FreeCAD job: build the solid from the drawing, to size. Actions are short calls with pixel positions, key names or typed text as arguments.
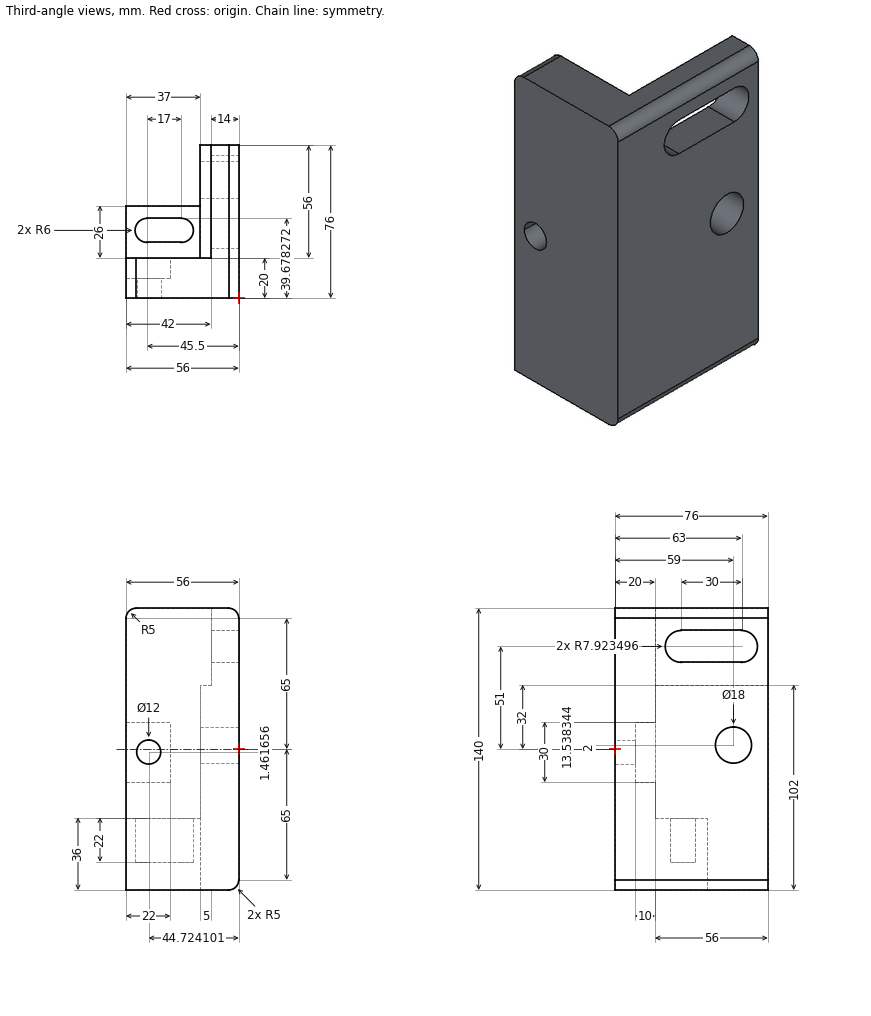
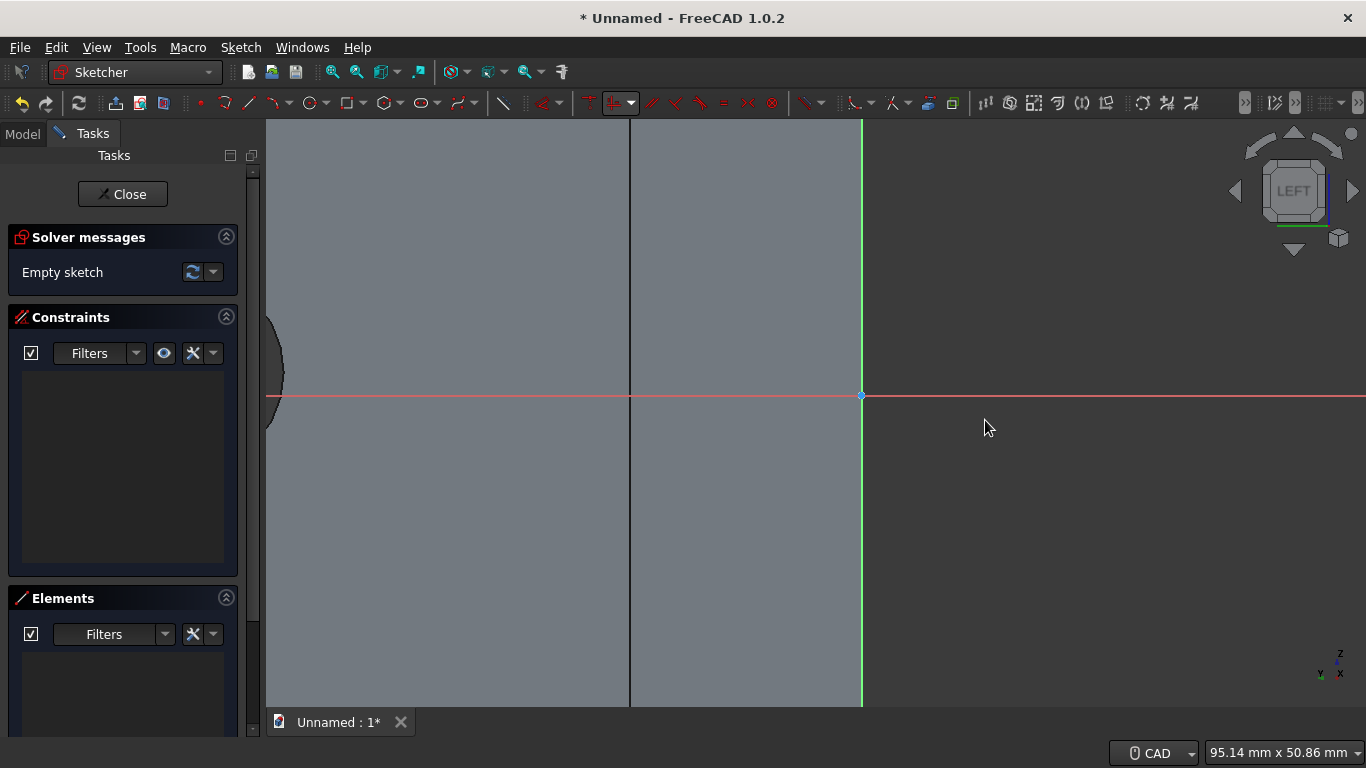
key(g)
key(r)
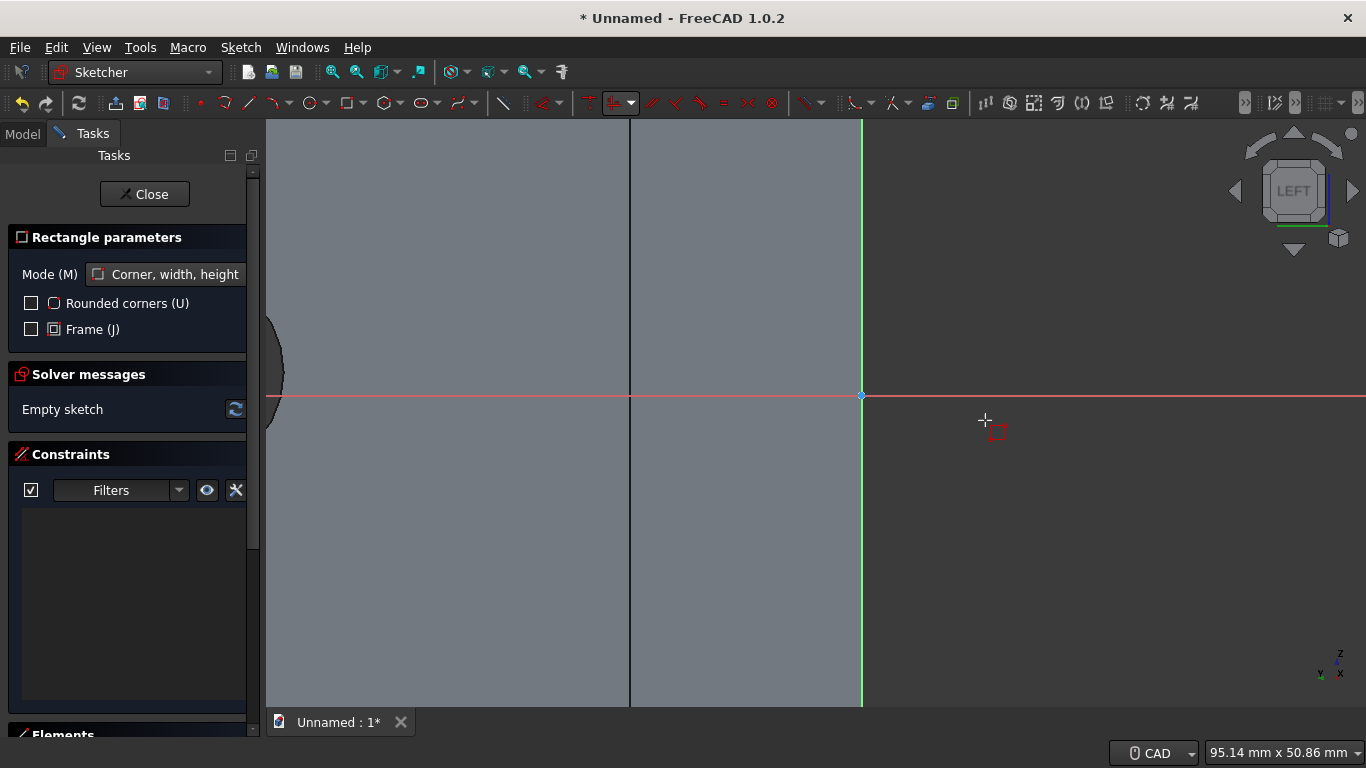
click(630, 239)
click(746, 586)
key(Escape)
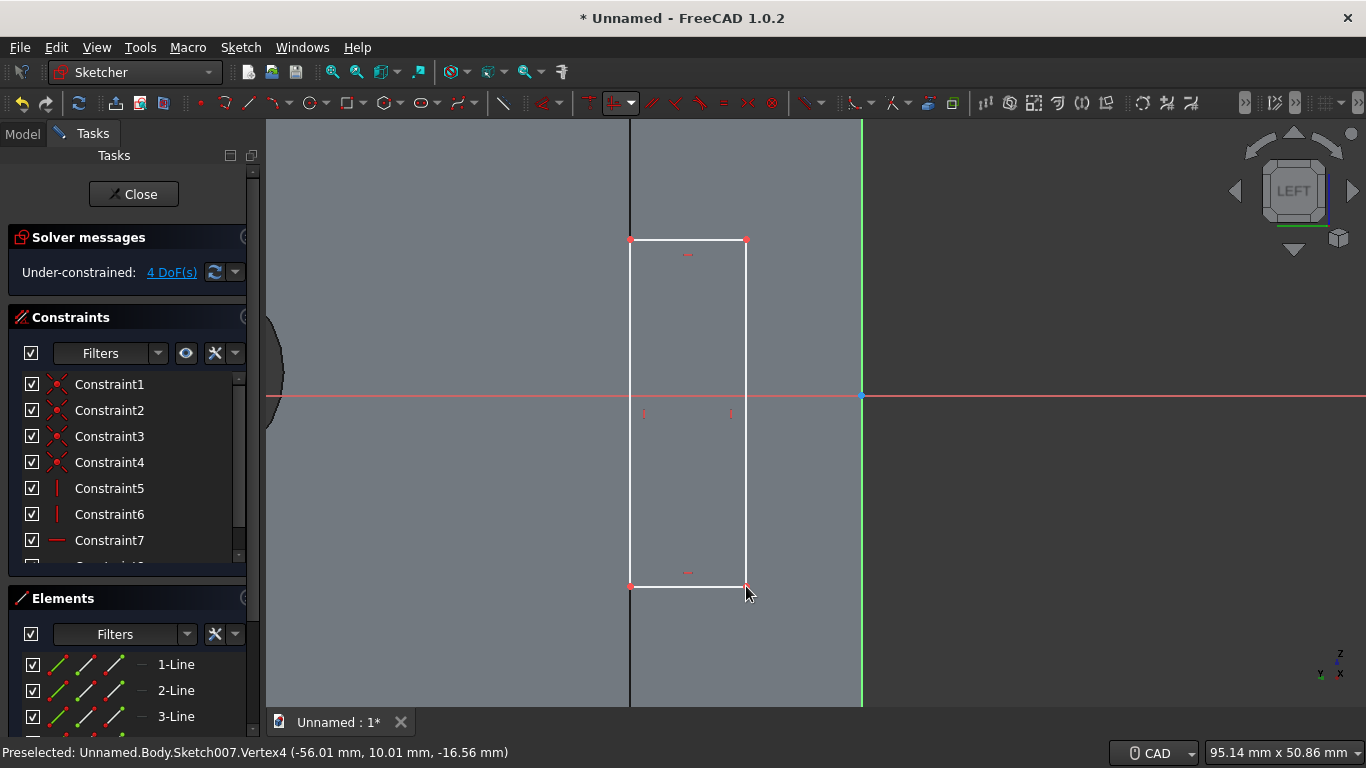
click(542, 104)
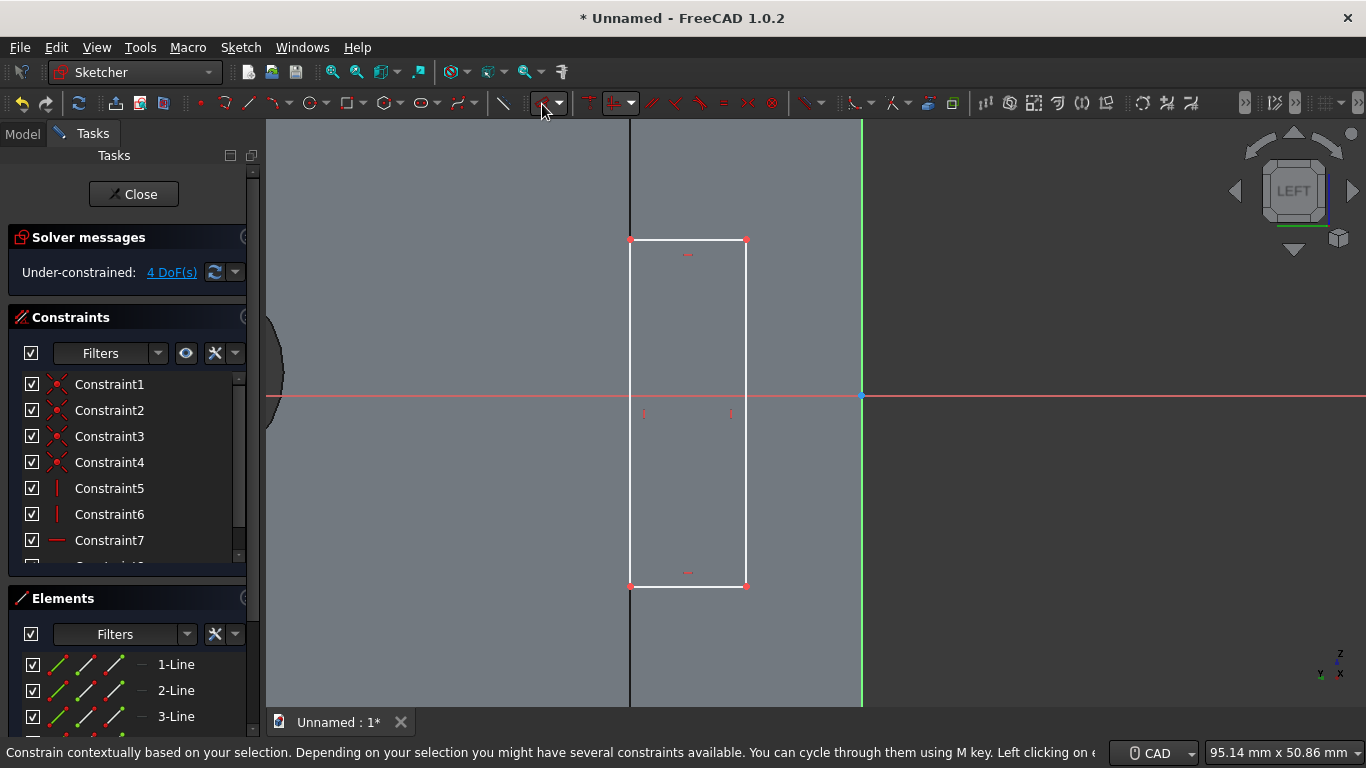
click(630, 344)
click(596, 413)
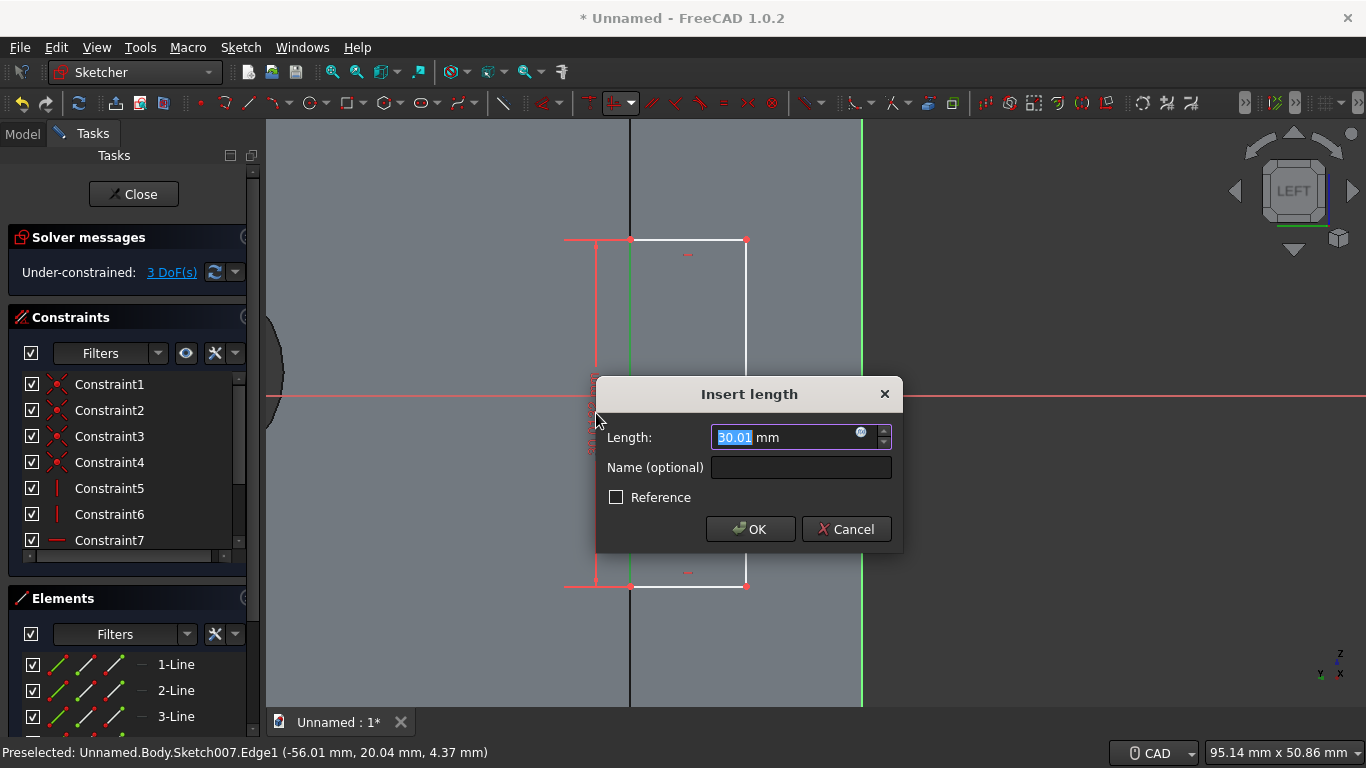
text(30)
key(Return)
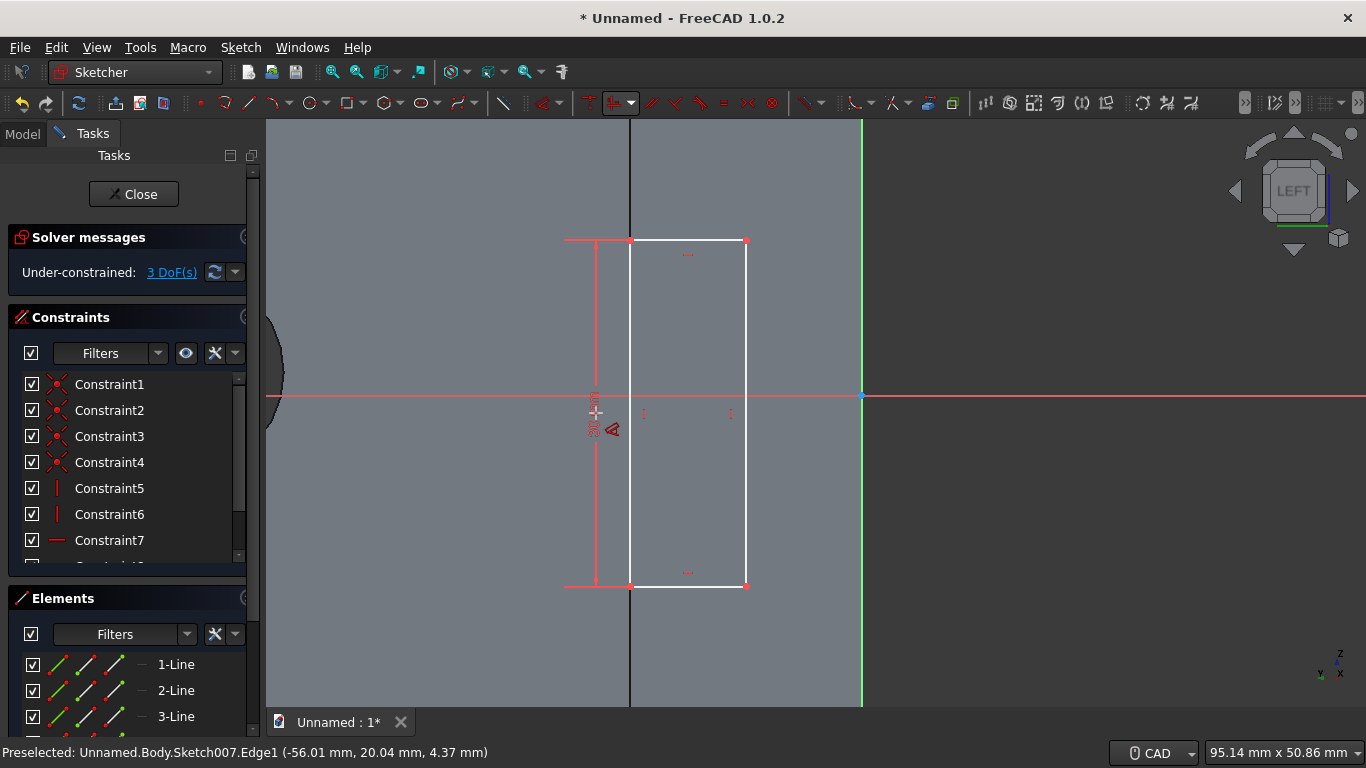
click(665, 587)
click(688, 621)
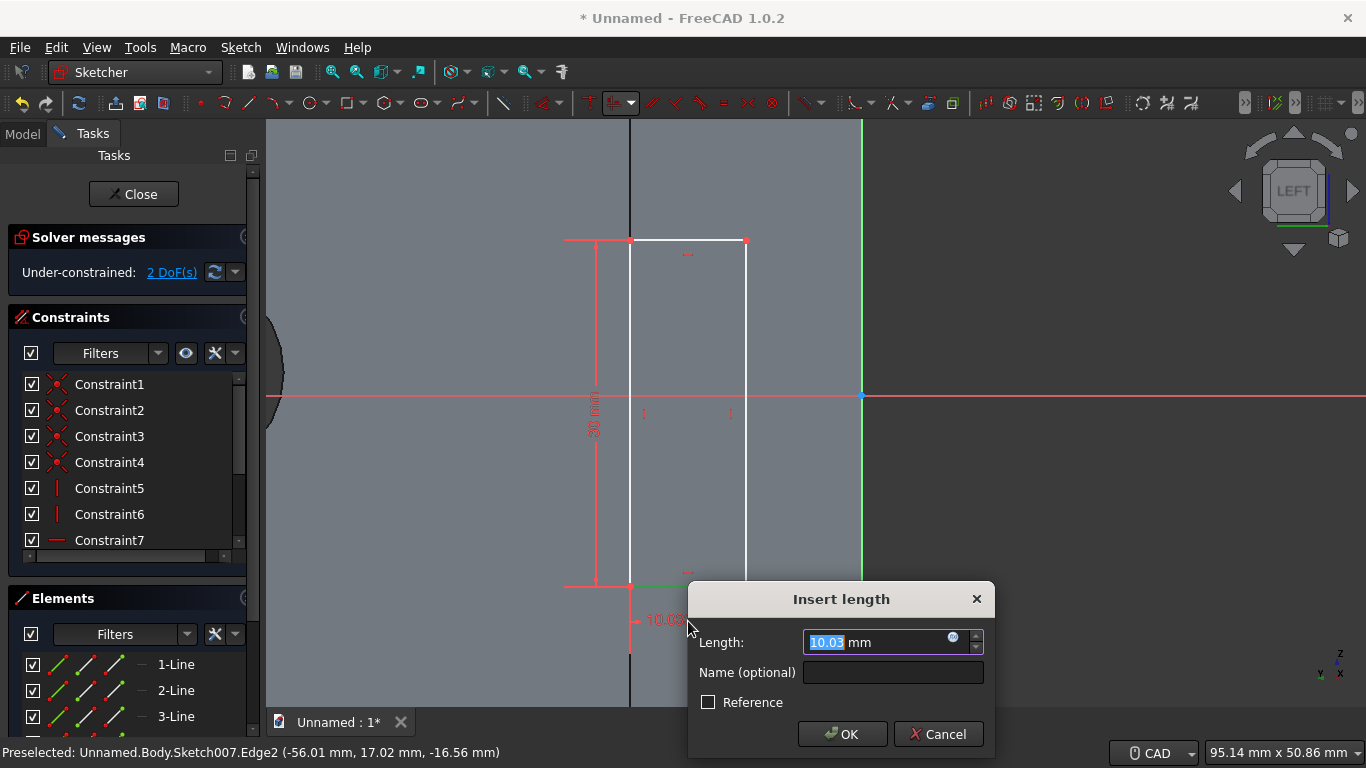
text(10)
key(Return)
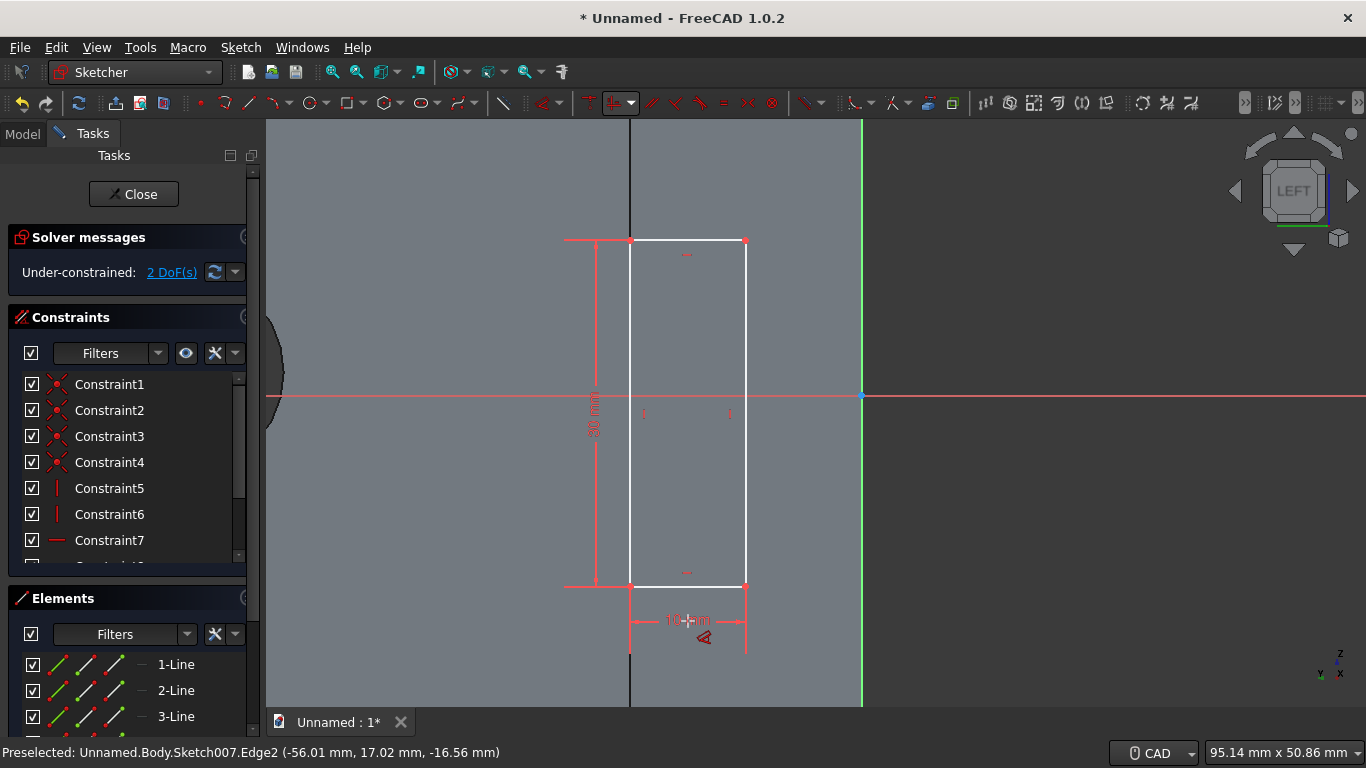
click(630, 240)
click(746, 206)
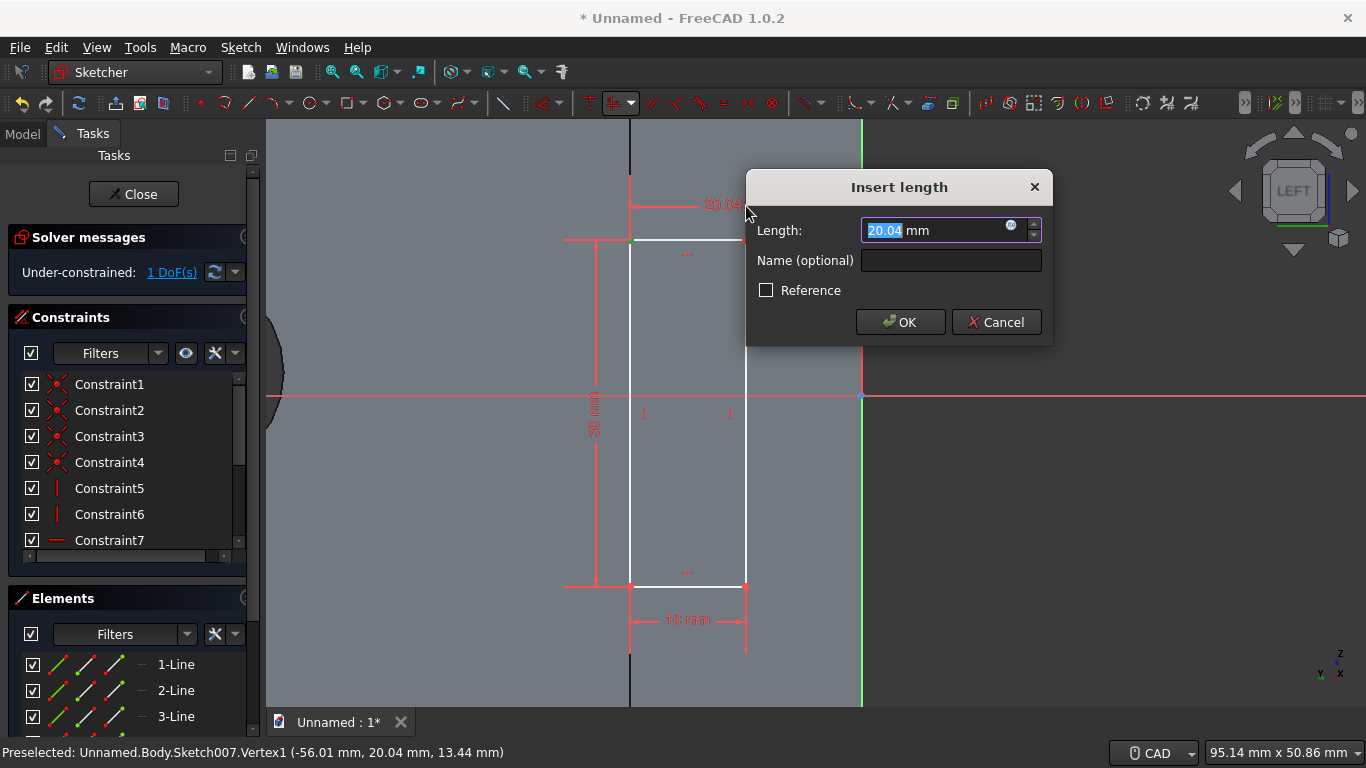
text(20)
key(Return)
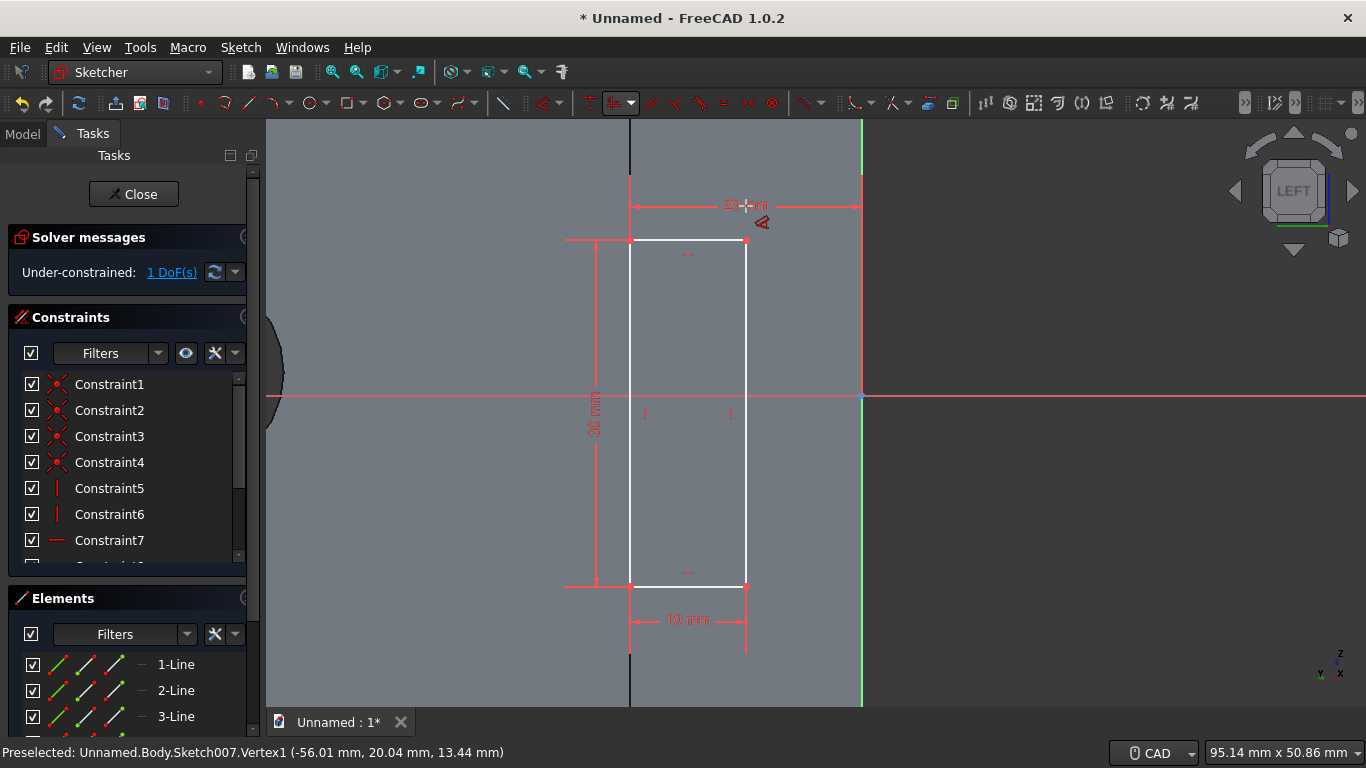
click(630, 240)
click(896, 318)